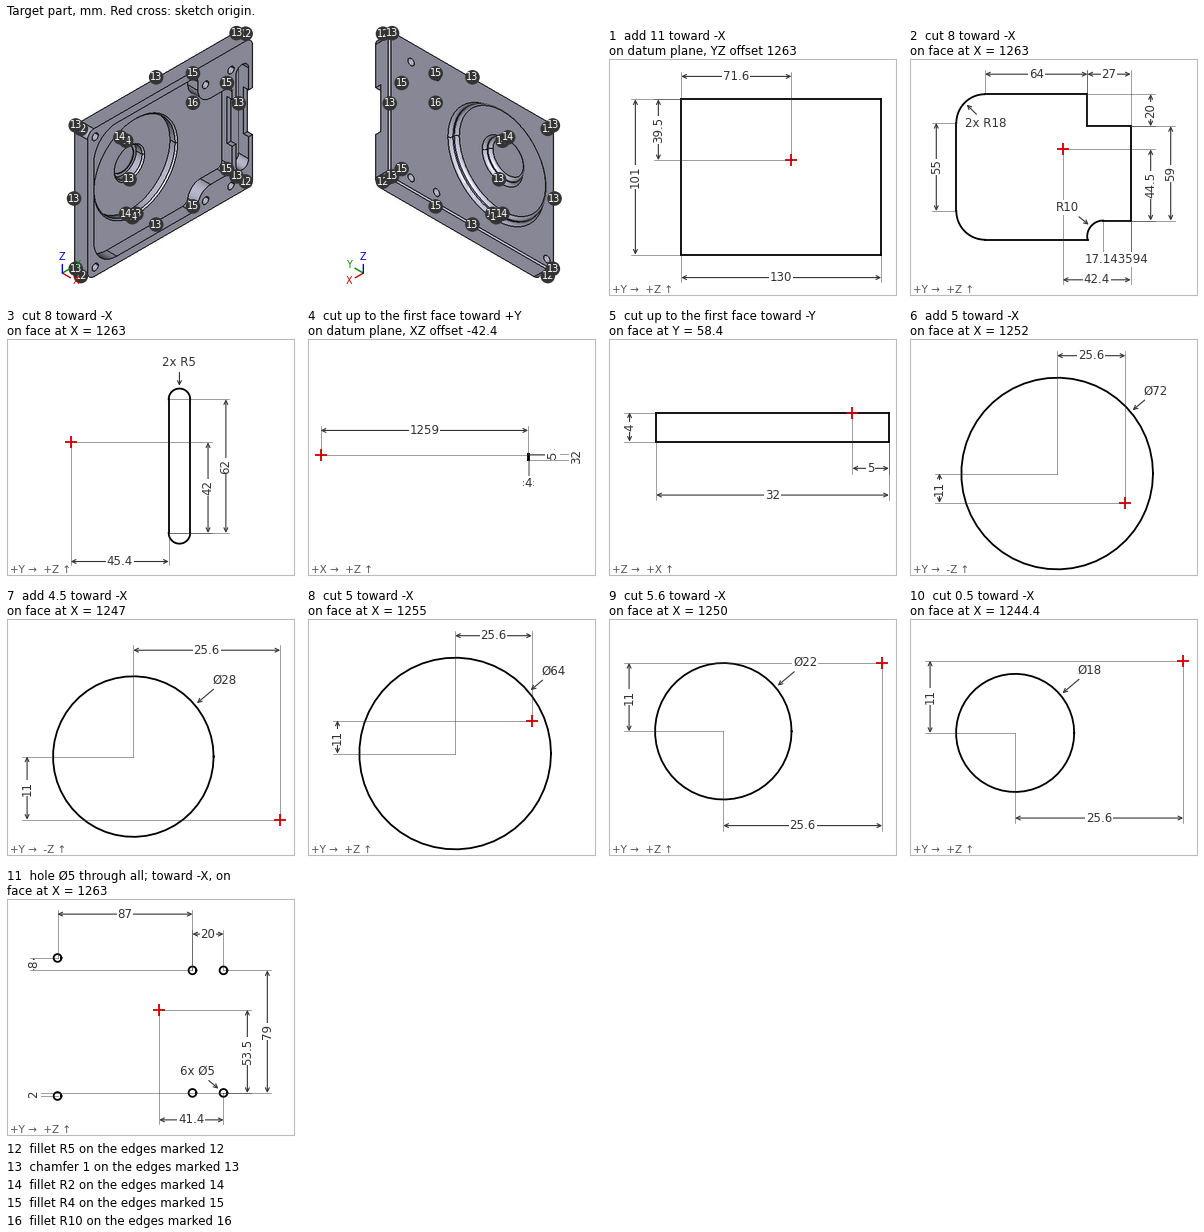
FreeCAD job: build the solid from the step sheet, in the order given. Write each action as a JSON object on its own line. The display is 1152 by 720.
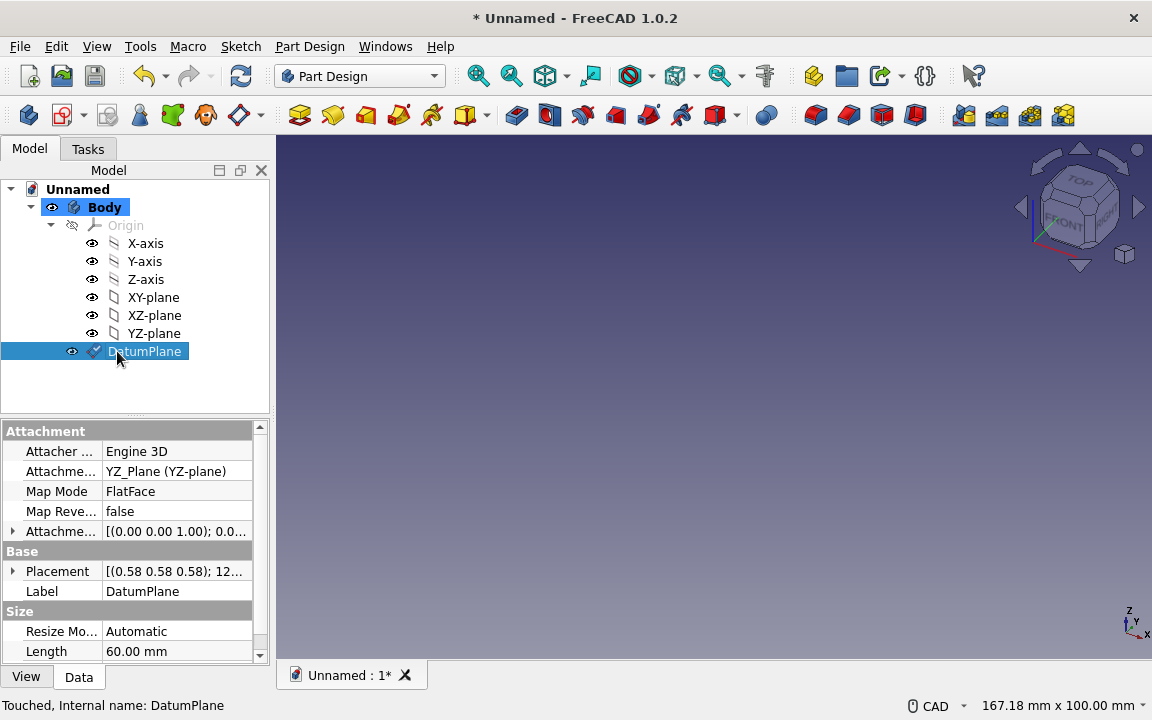
{"action": "left_click", "coordinate": [62, 116]}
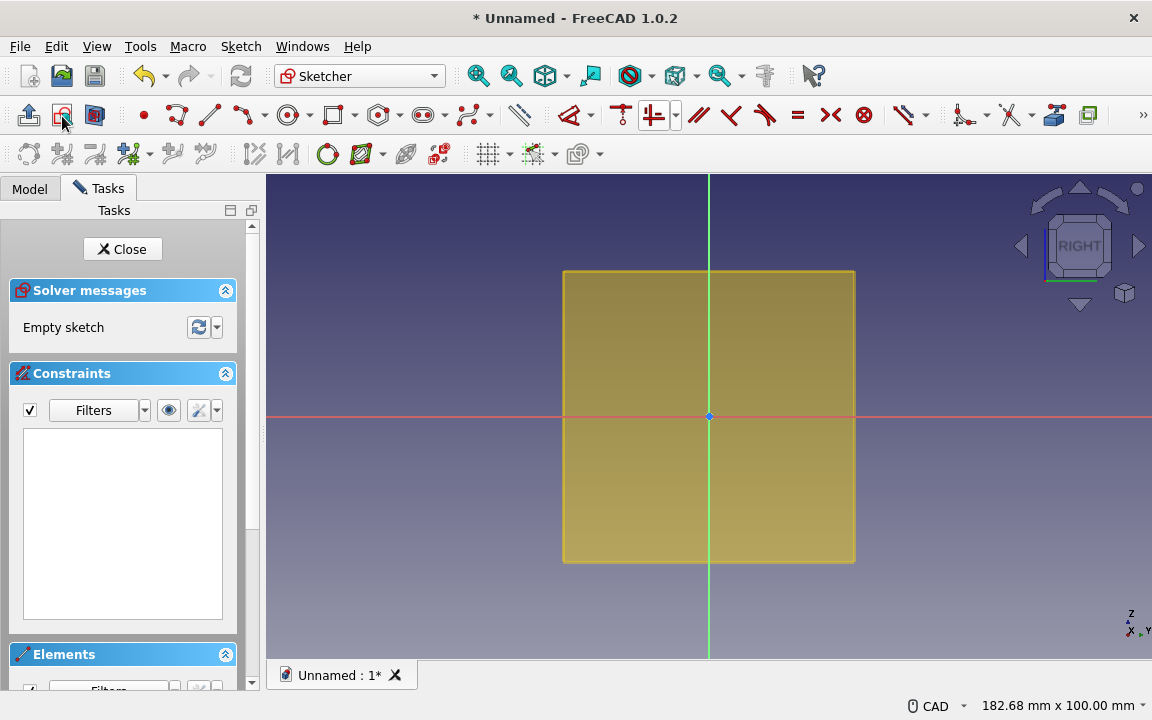
{"action": "scroll", "coordinate": [566, 308], "scroll_direction": "down", "scroll_amount": 2}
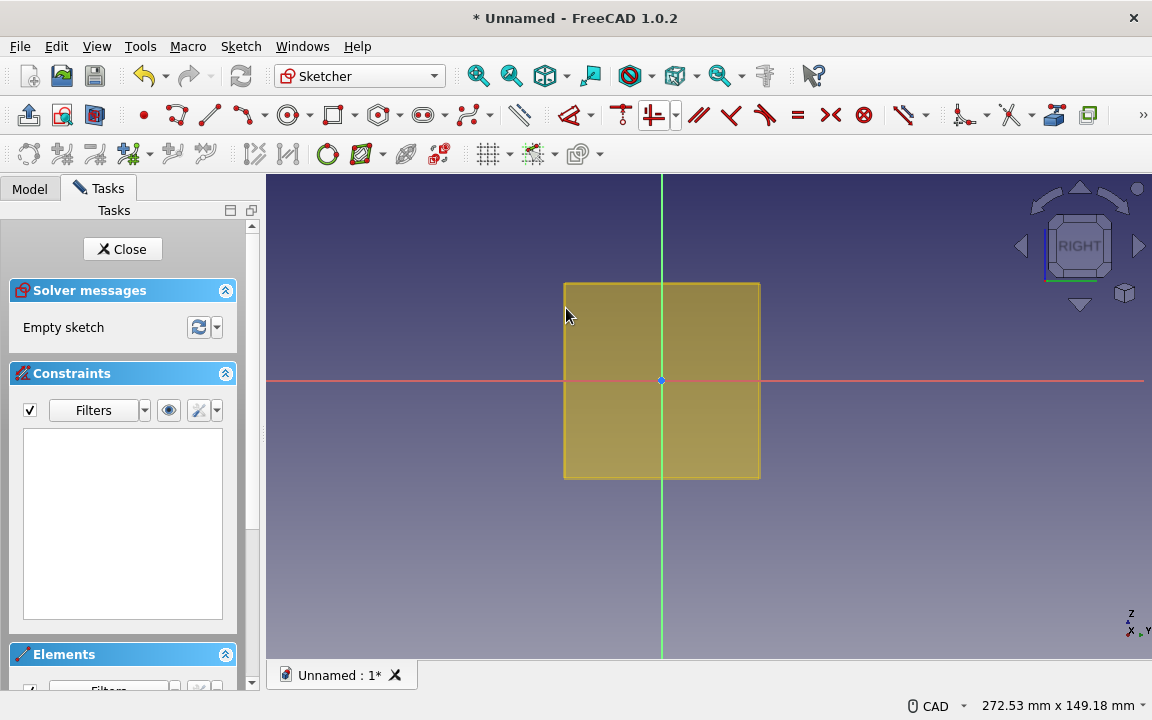
{"action": "left_click", "coordinate": [332, 116]}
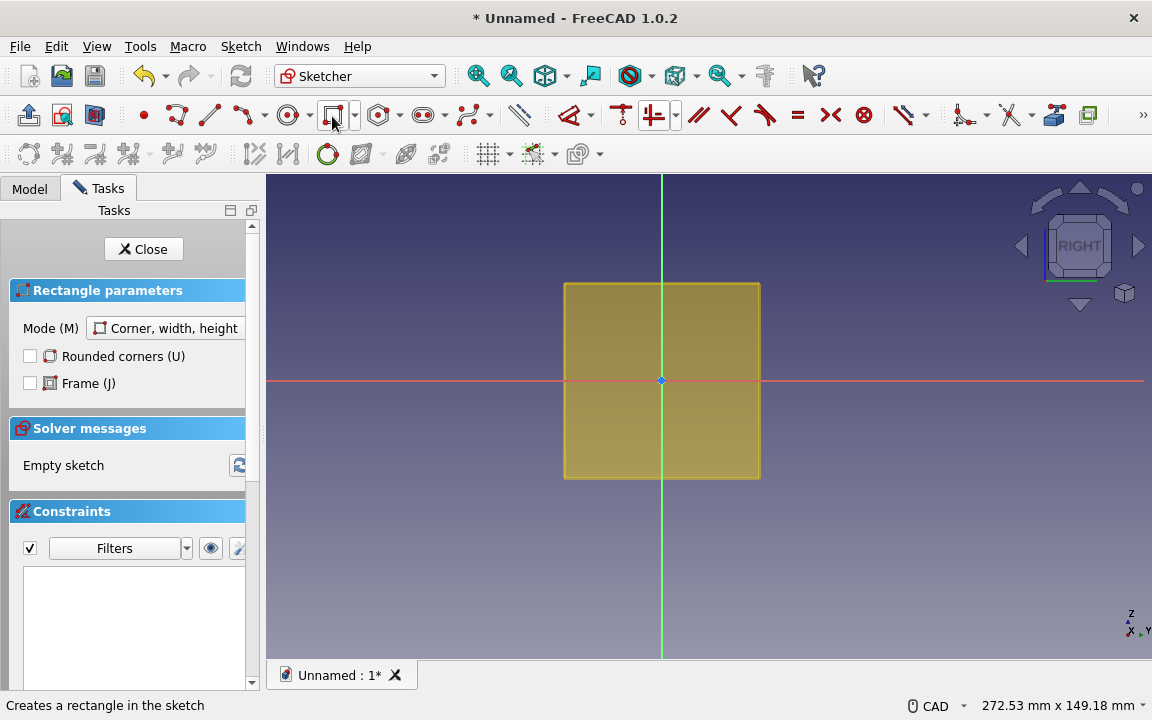
{"action": "left_click", "coordinate": [429, 252]}
{"action": "left_click", "coordinate": [852, 581]}
{"action": "key", "text": "Escape"}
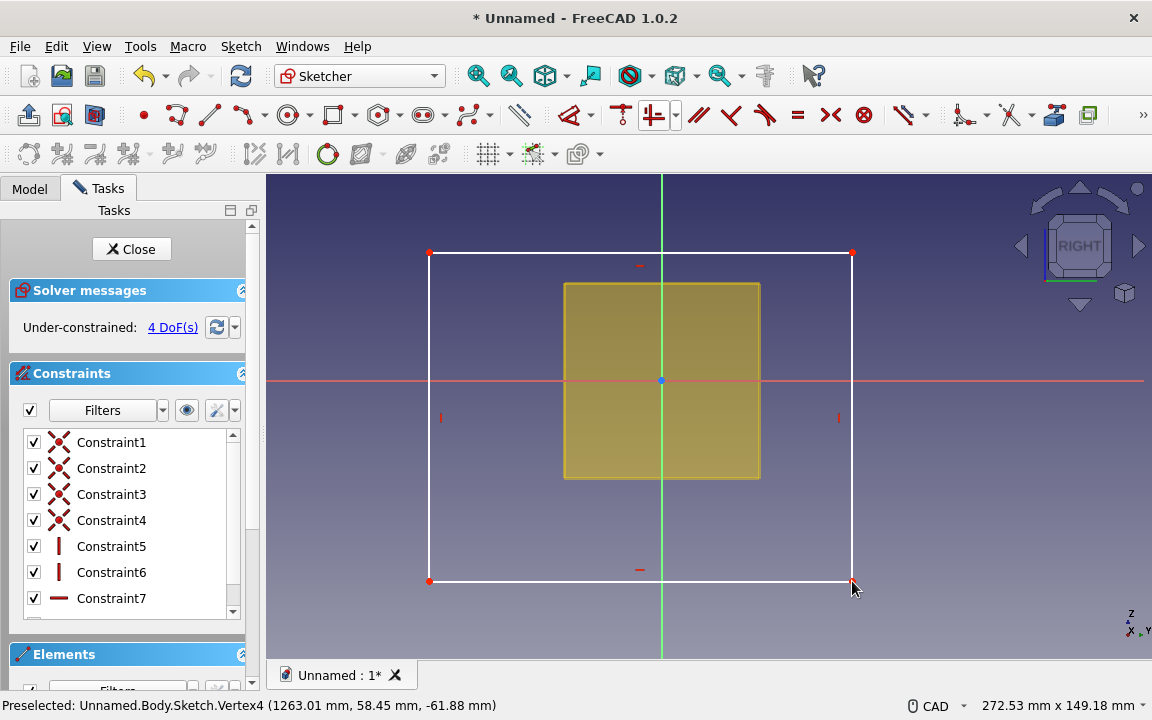
{"action": "left_click", "coordinate": [429, 352]}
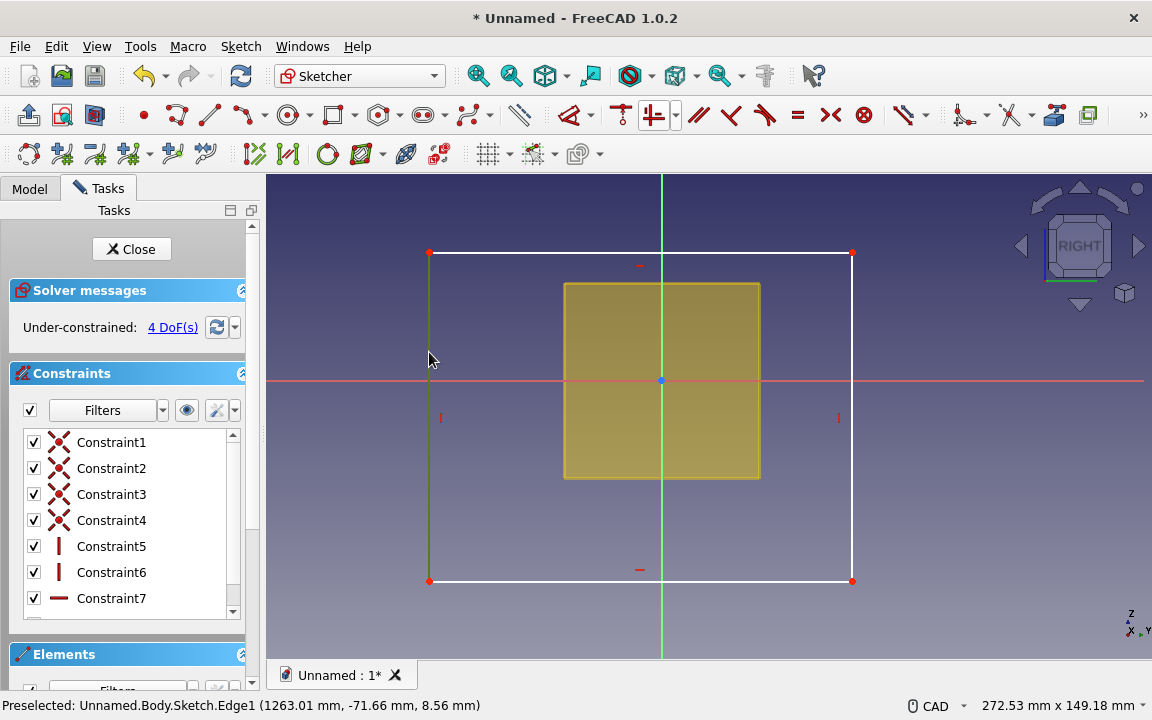
{"action": "key", "text": "i"}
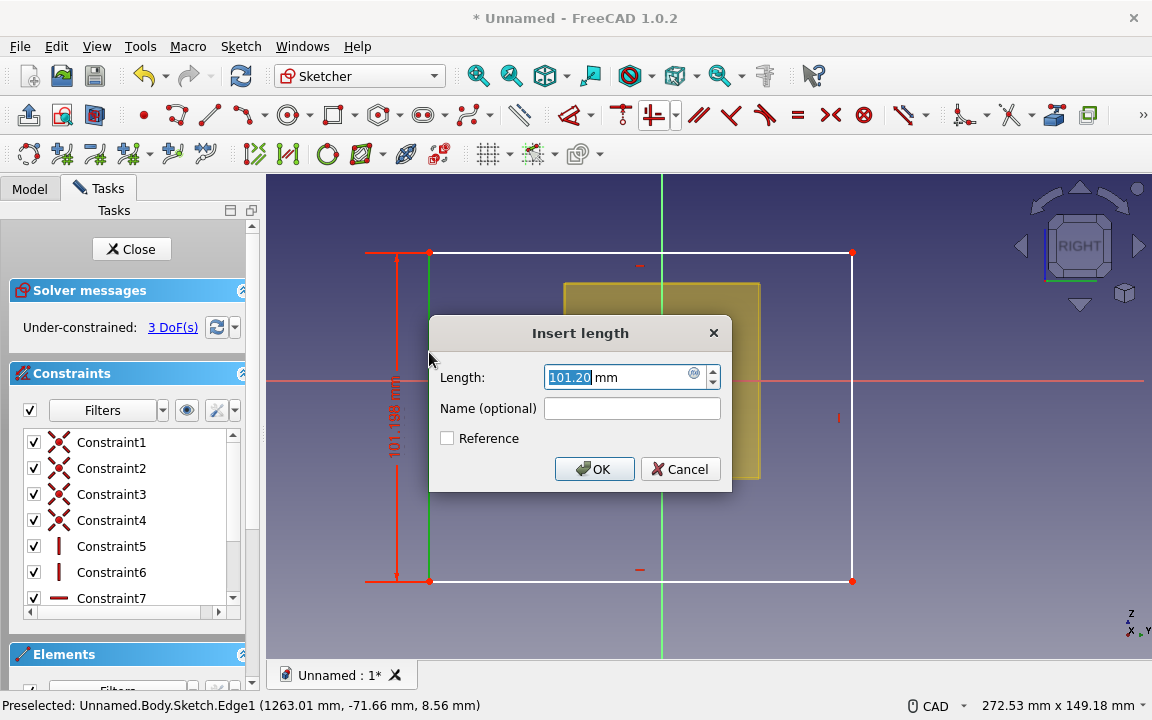
{"action": "type", "text": "101"}
{"action": "key", "text": "Return"}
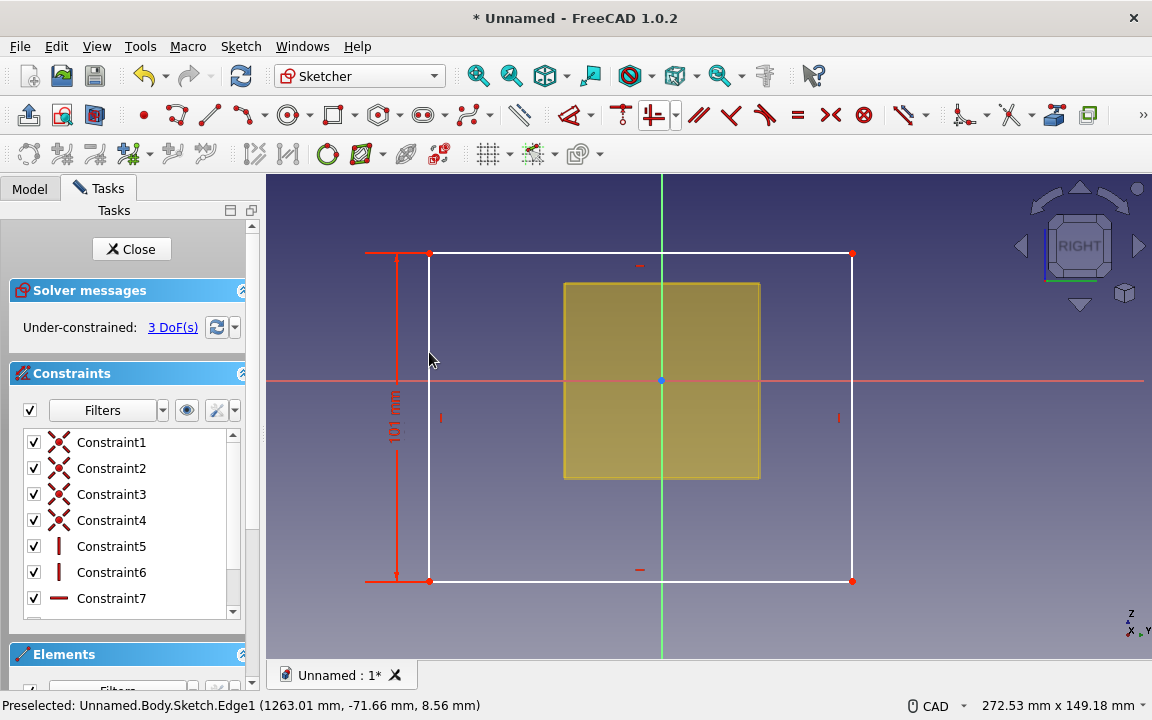
{"action": "left_click", "coordinate": [556, 582]}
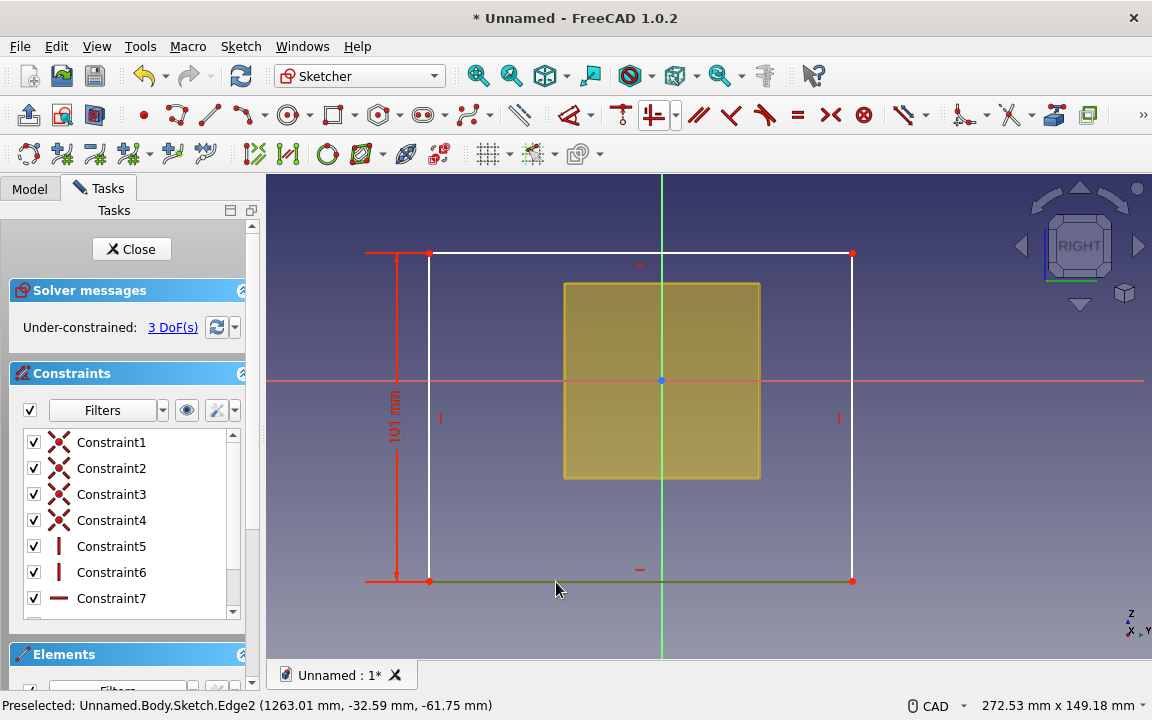
{"action": "left_click", "coordinate": [590, 116]}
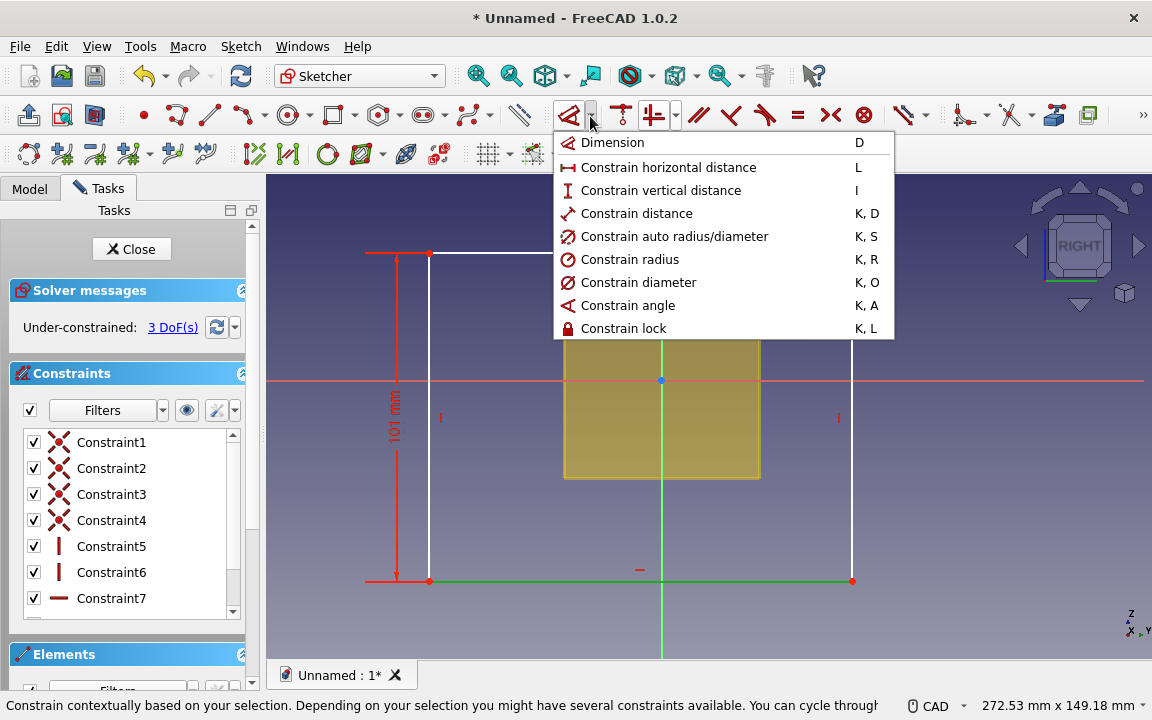
{"action": "left_click", "coordinate": [724, 168]}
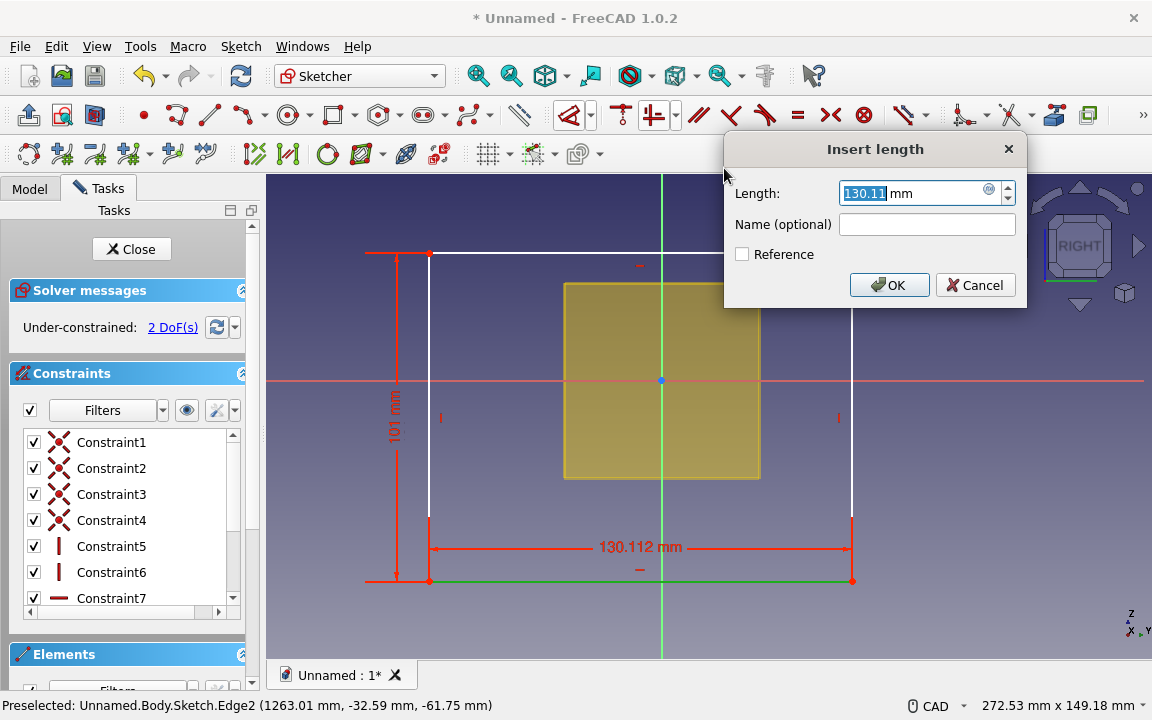
{"action": "type", "text": "130"}
{"action": "key", "text": "Return"}